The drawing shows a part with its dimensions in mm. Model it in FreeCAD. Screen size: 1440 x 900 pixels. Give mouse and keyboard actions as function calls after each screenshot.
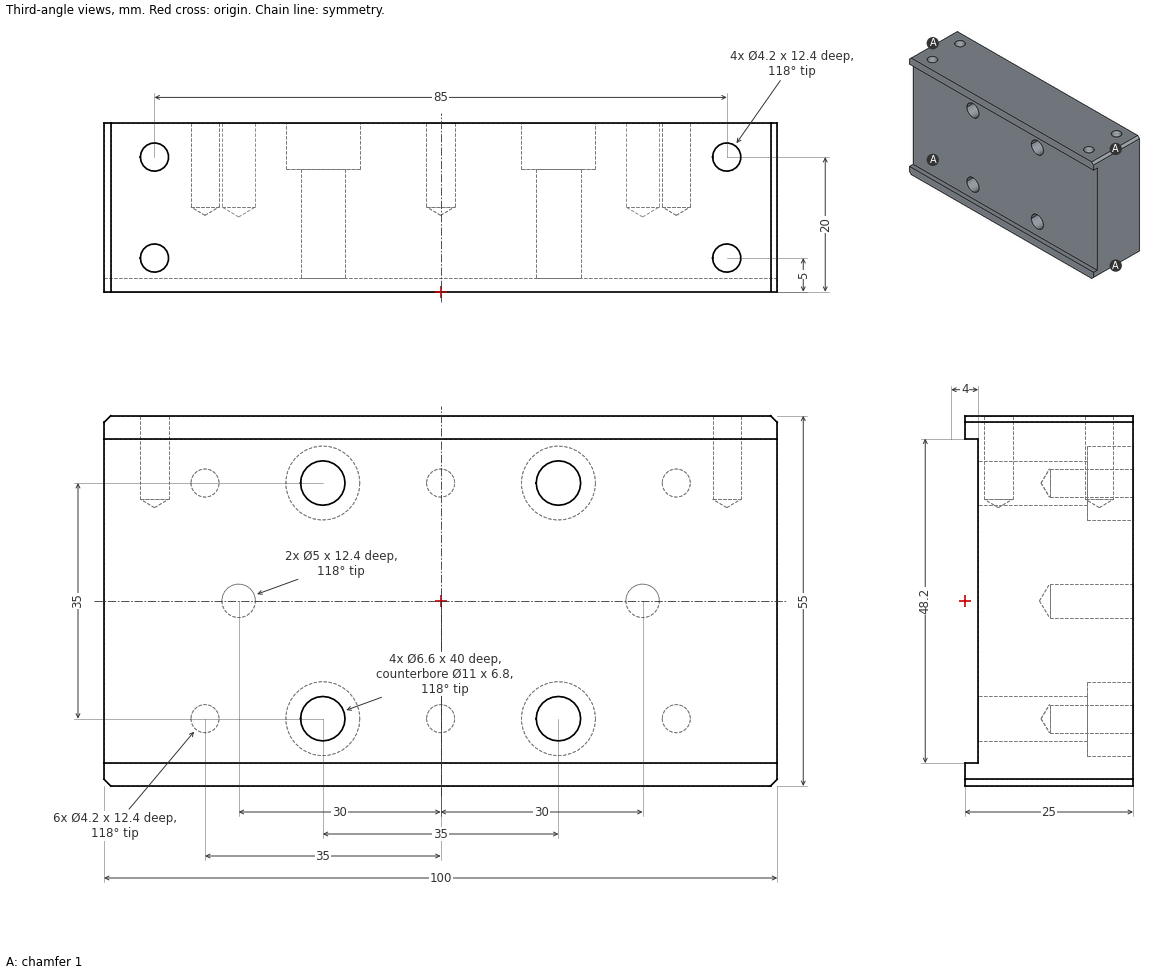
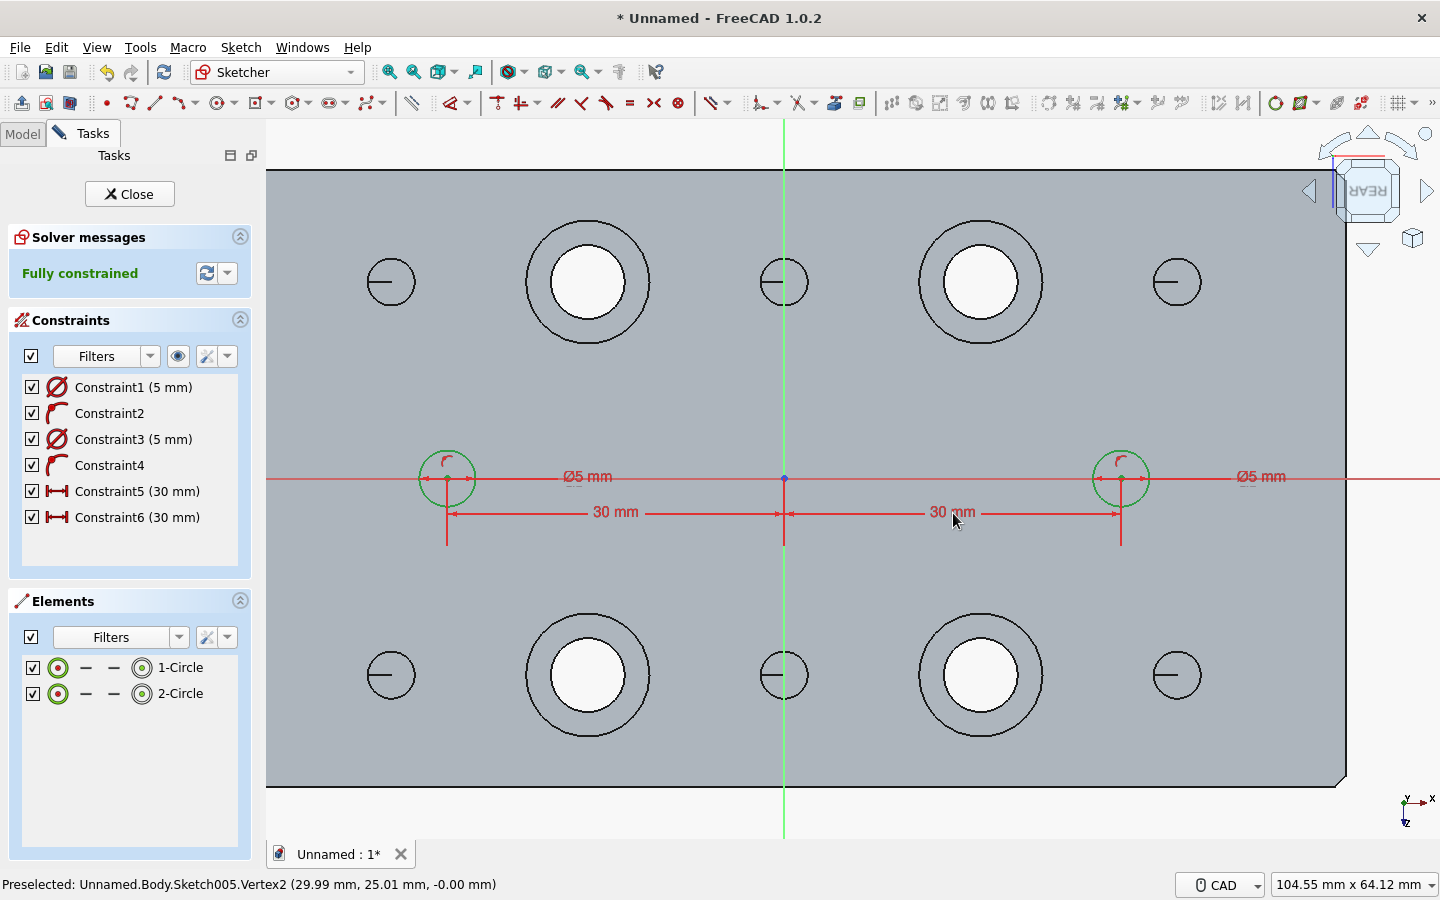
click(130, 194)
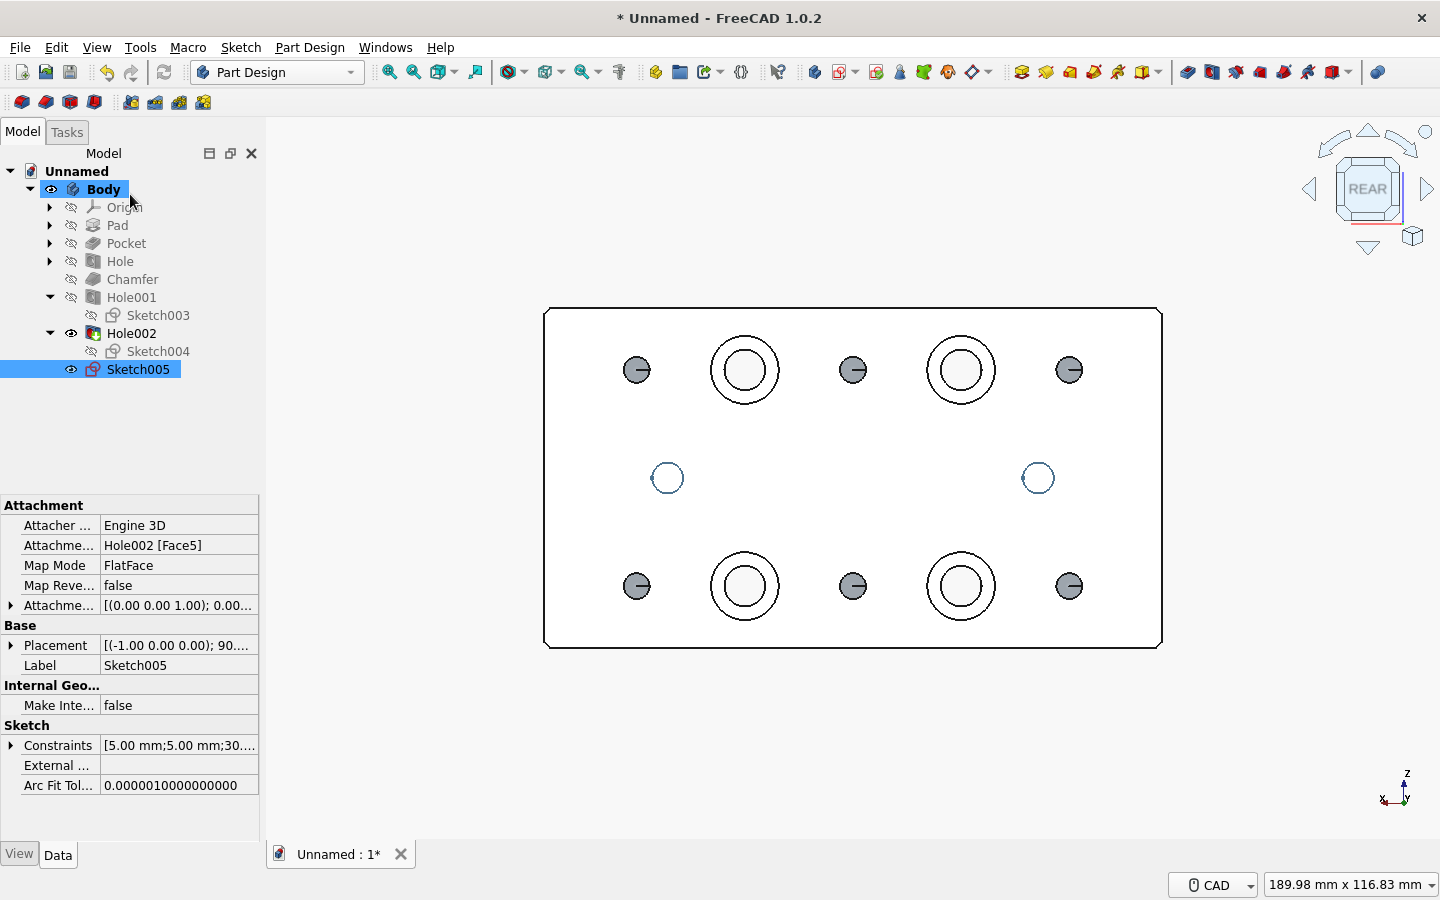
click(1212, 72)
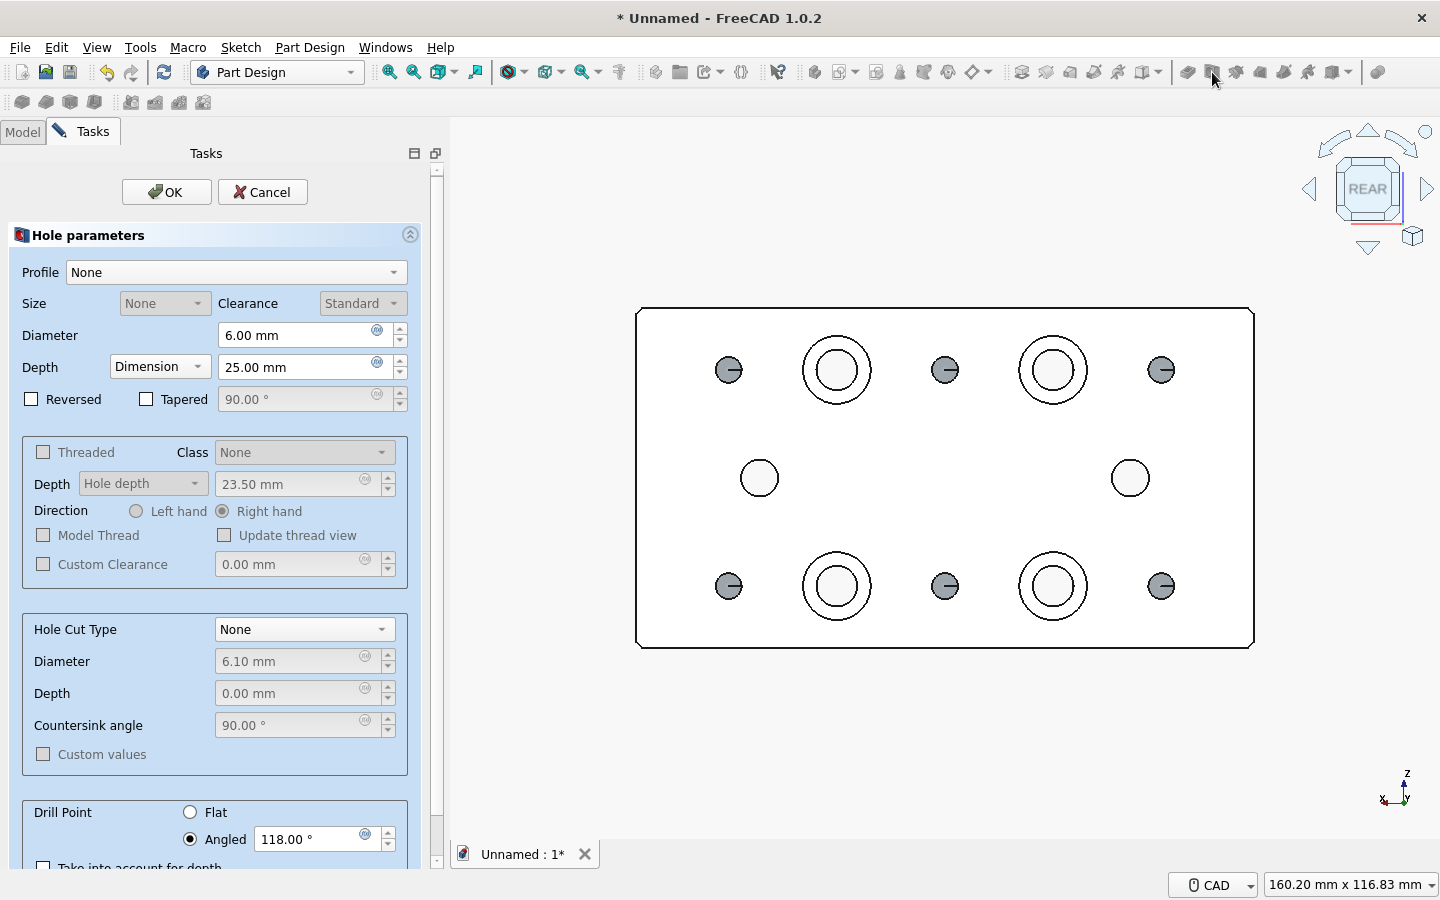
triple_click(305, 335)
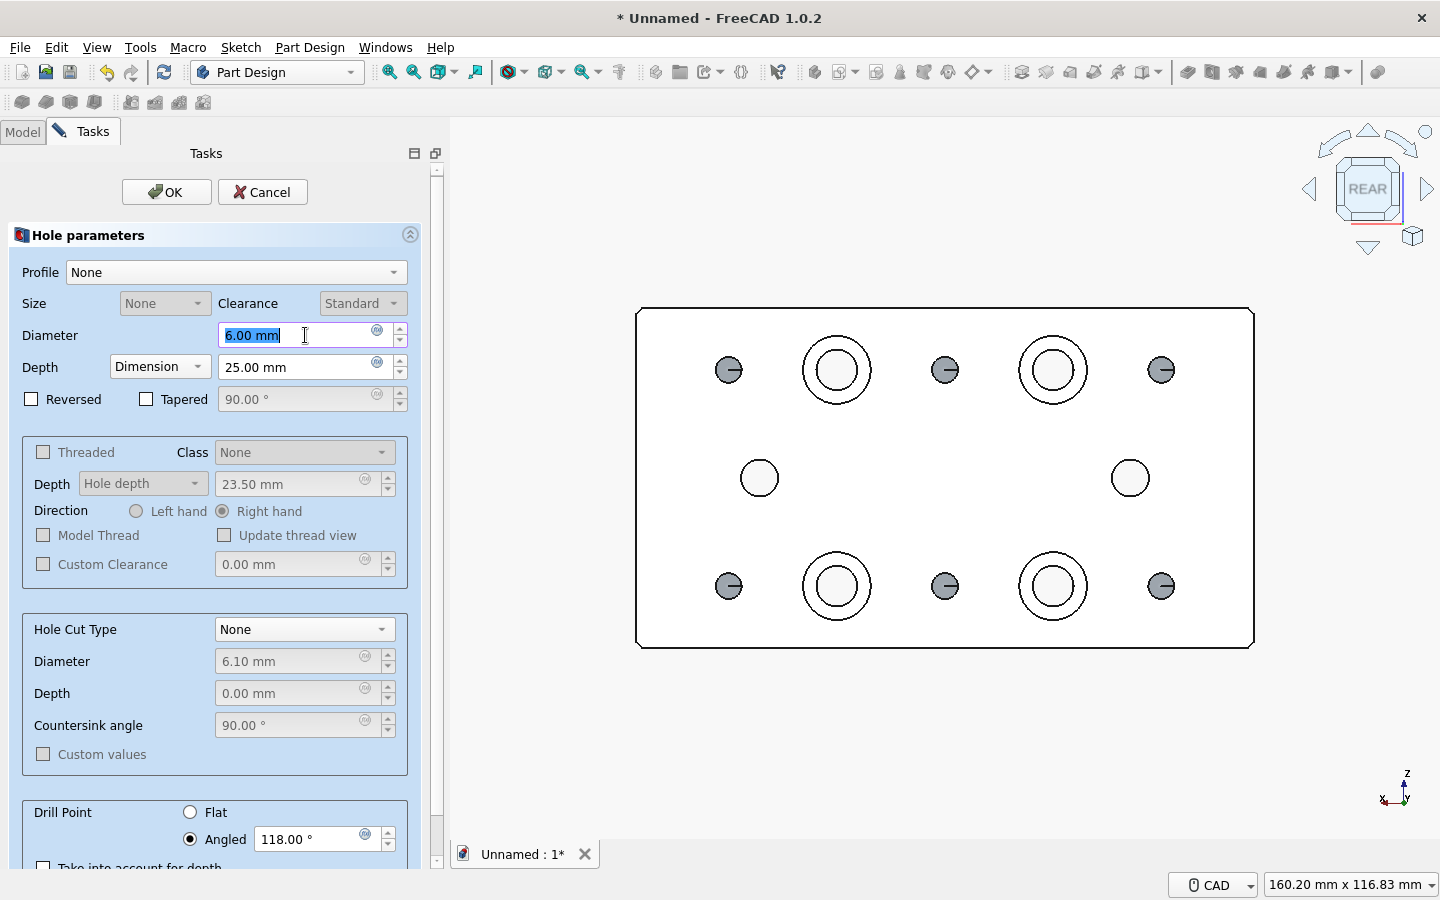
text(5)
key(Tab)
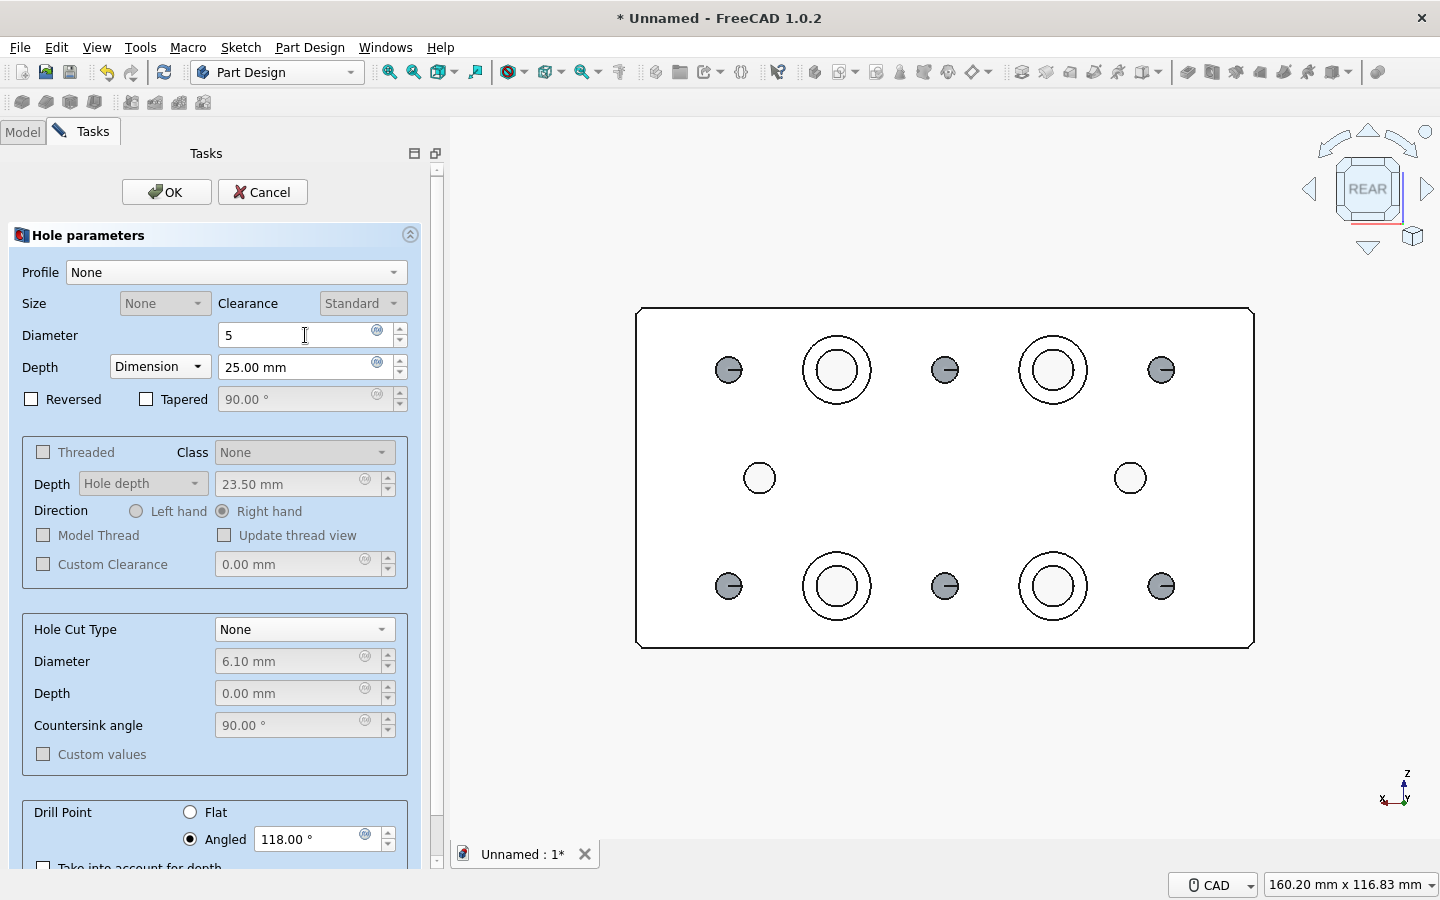
triple_click(305, 367)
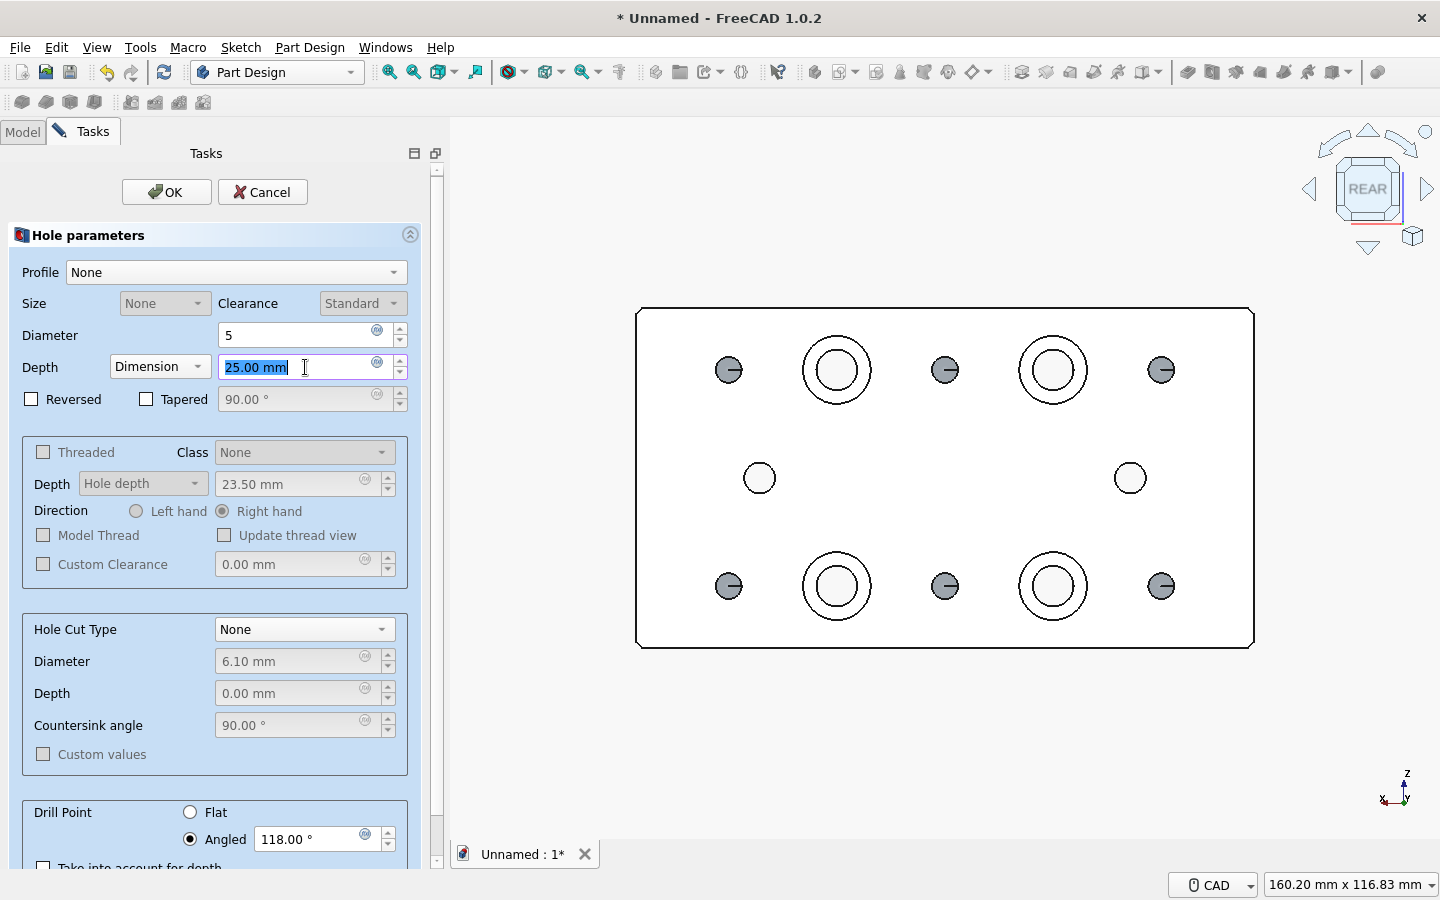
text(12.4)
key(Tab)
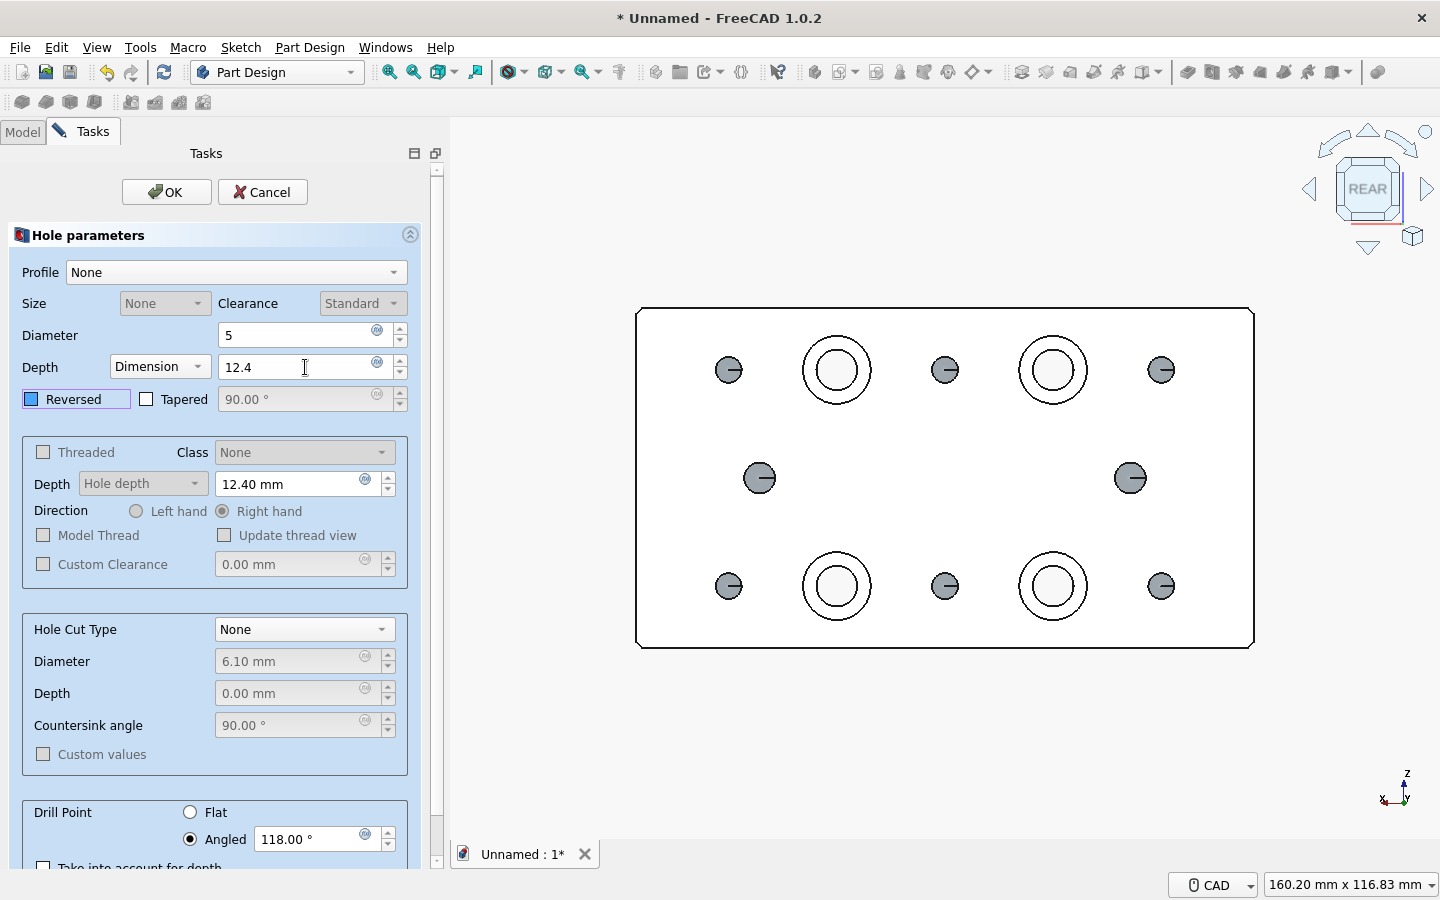
click(167, 192)